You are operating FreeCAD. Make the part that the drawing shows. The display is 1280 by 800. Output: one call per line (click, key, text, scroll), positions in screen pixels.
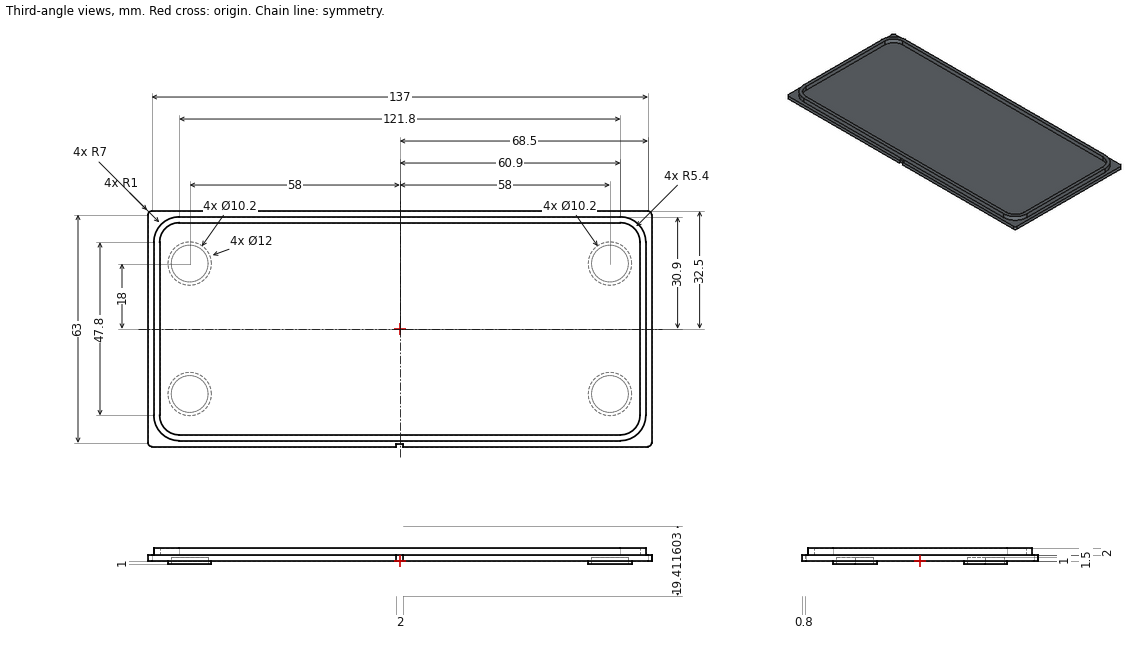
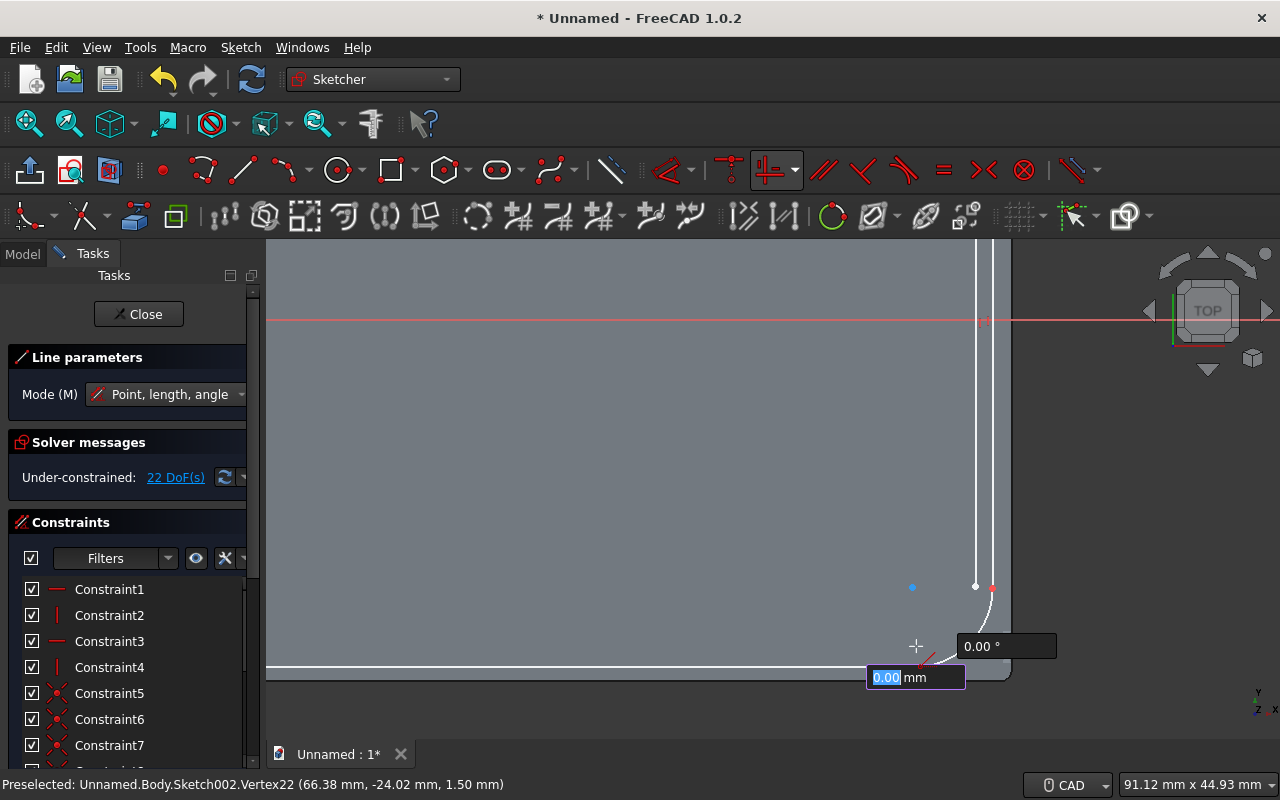
scroll(976, 588, down, 5)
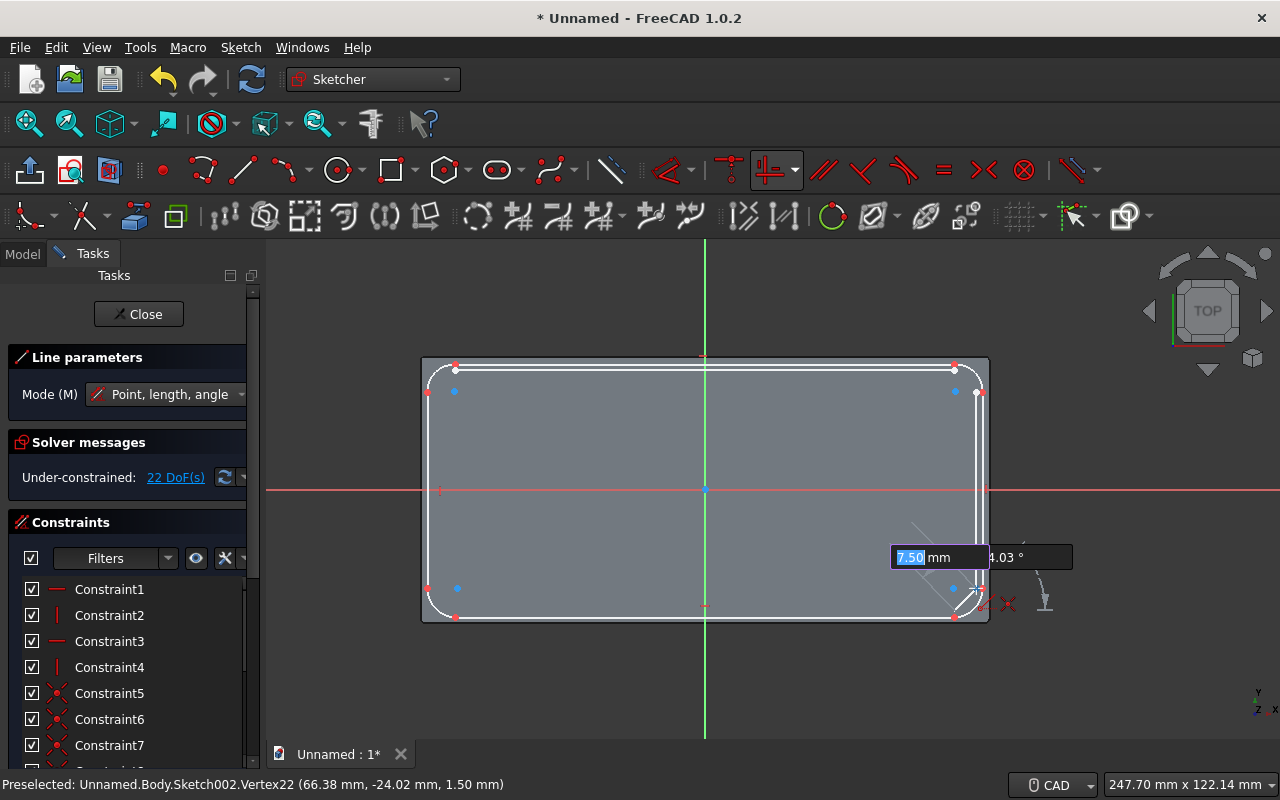
scroll(456, 610, up, 5)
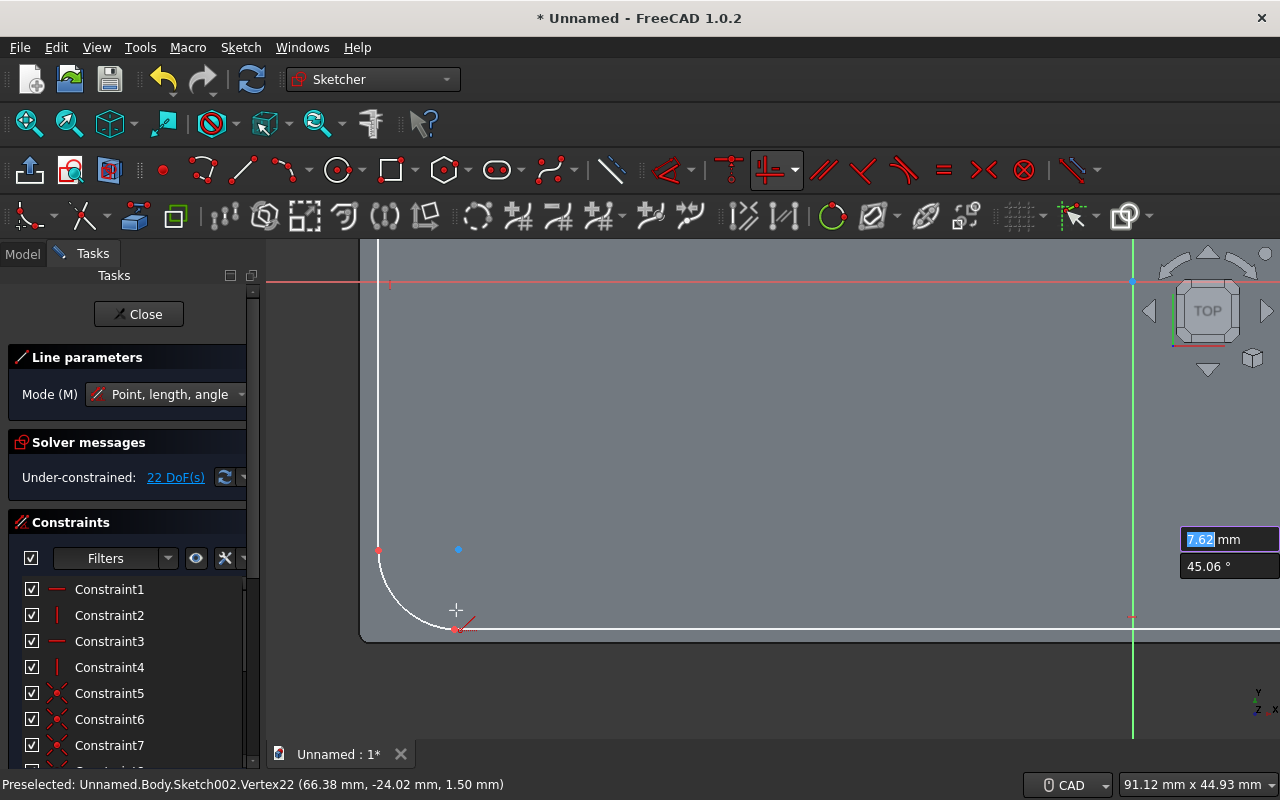
click(455, 608)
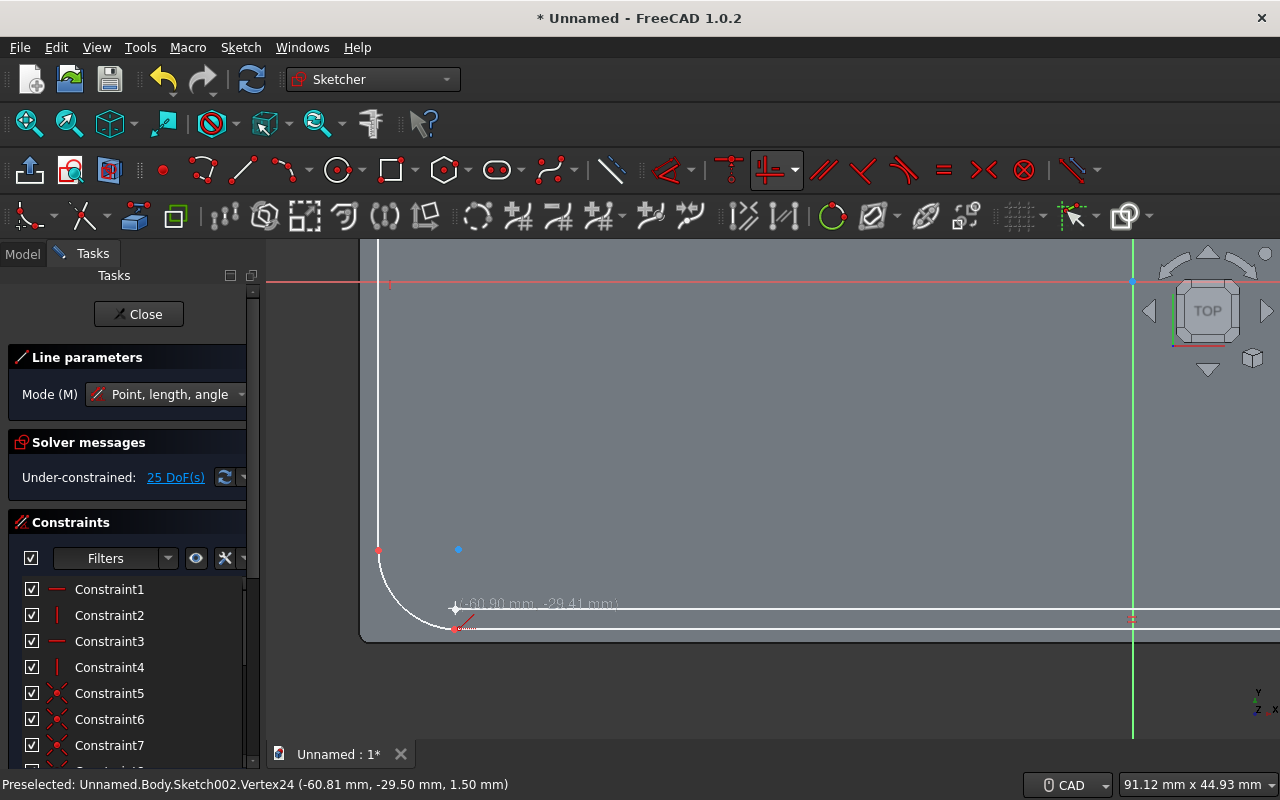
click(395, 548)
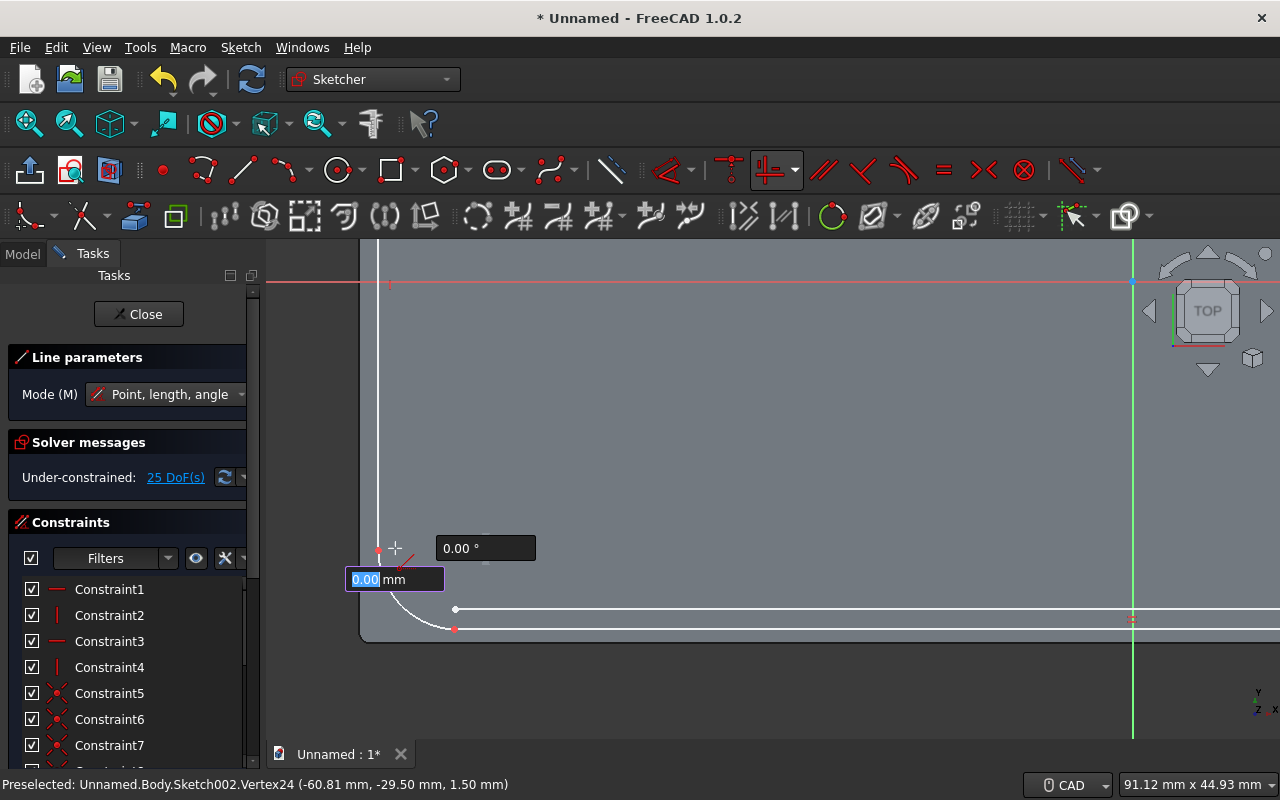
scroll(455, 610, down, 5)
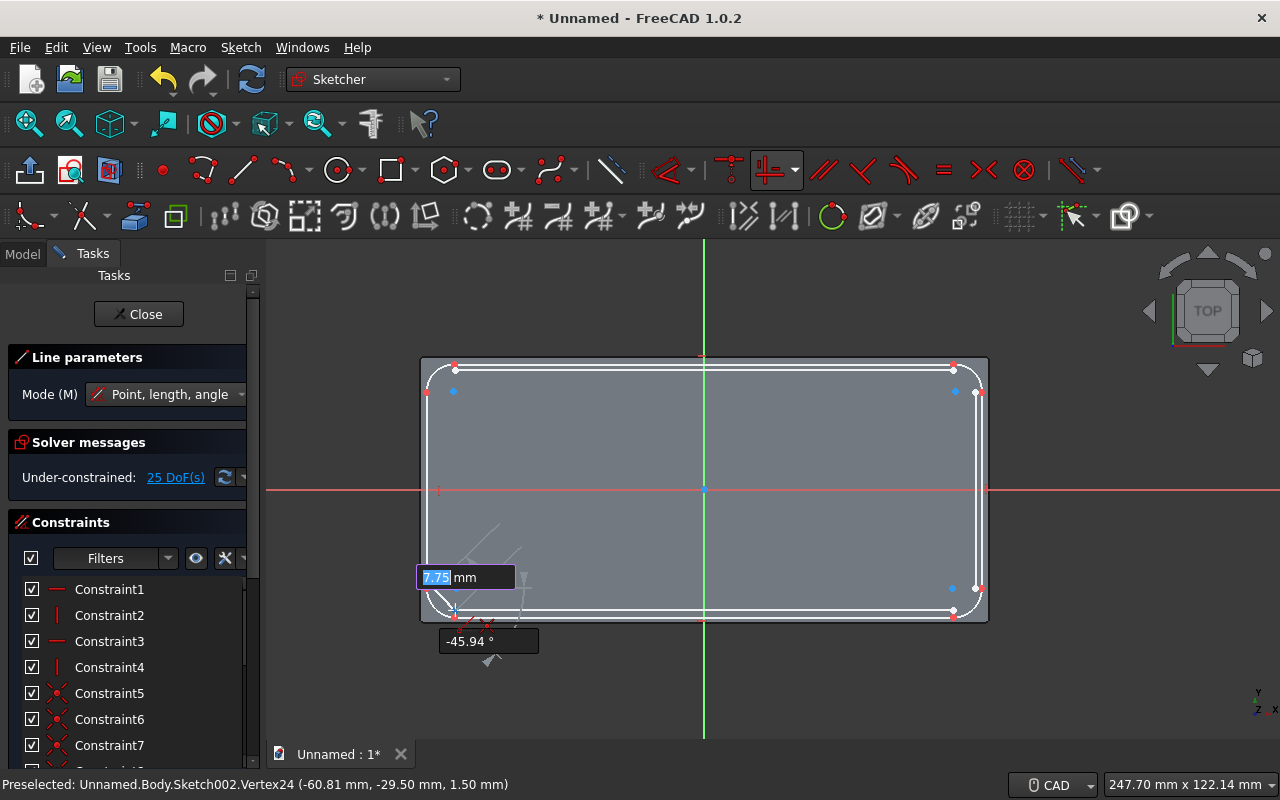
scroll(433, 392, up, 5)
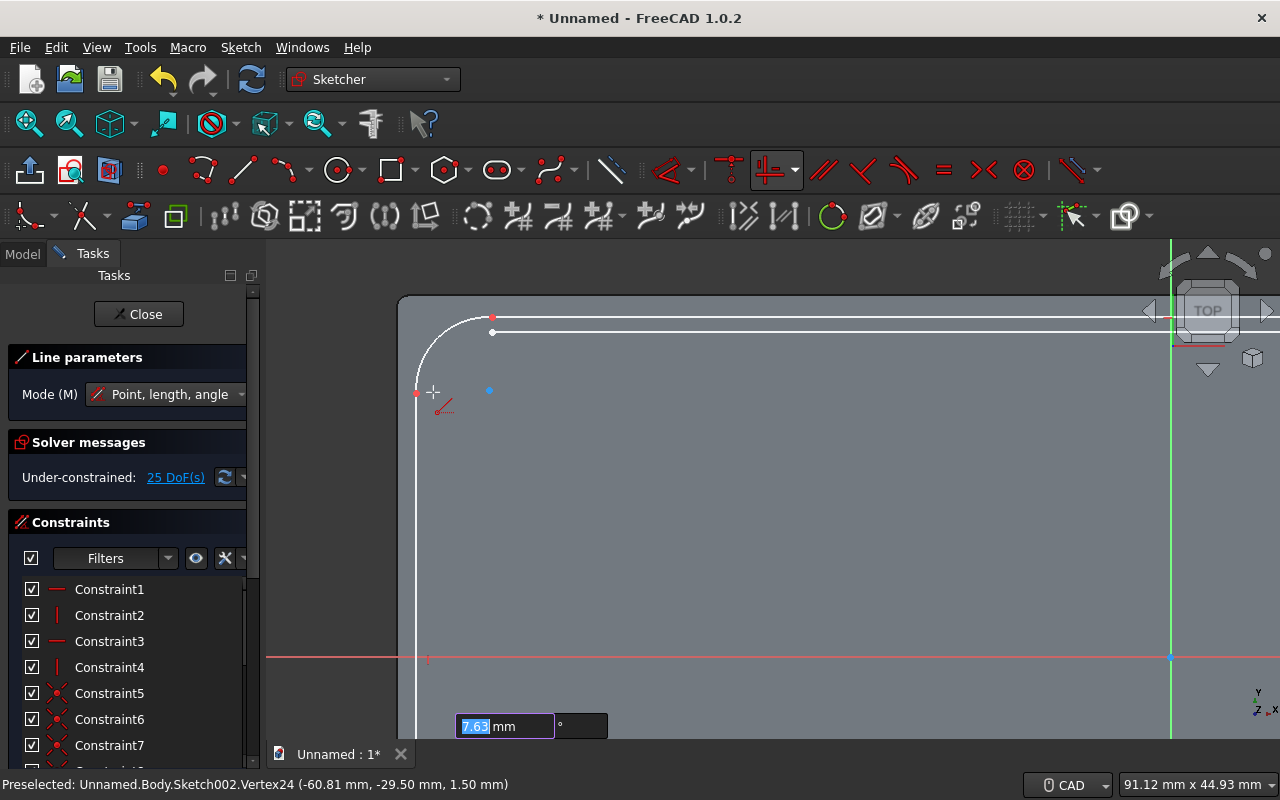
click(433, 391)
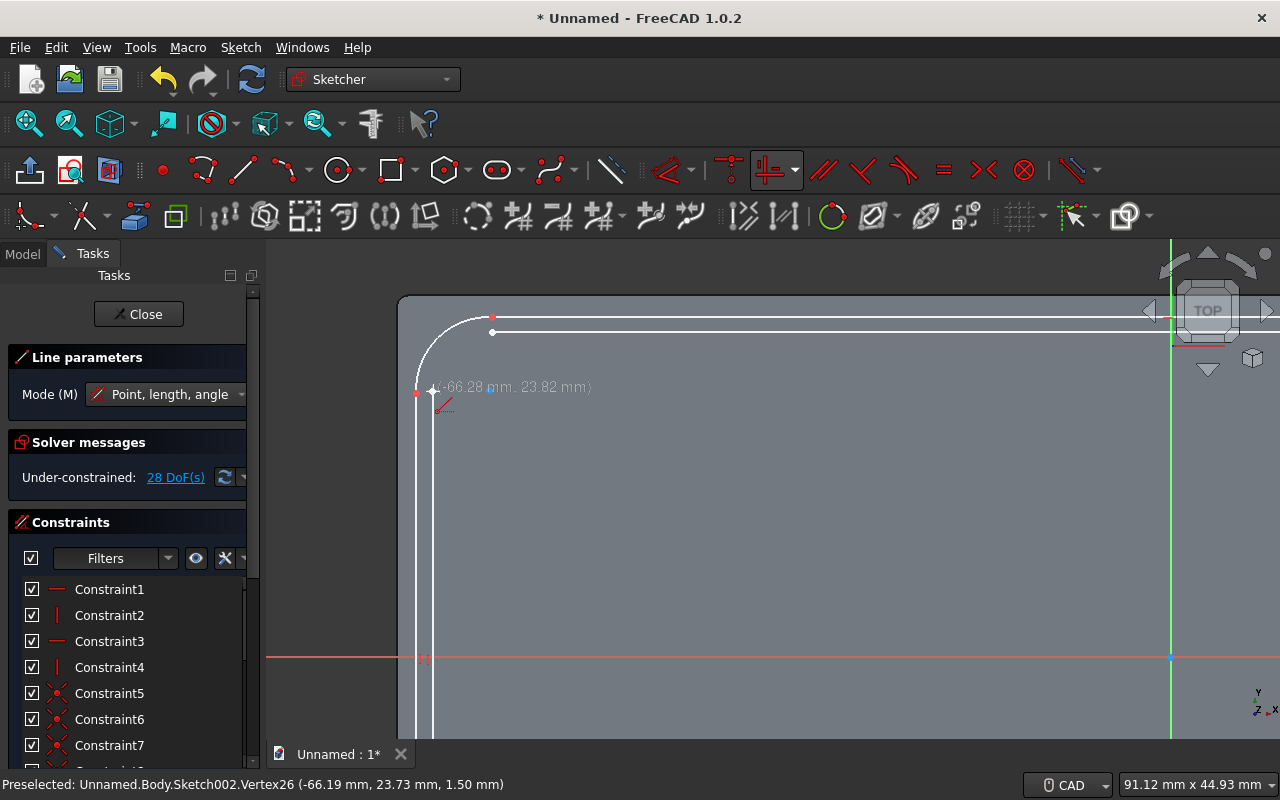
click(284, 170)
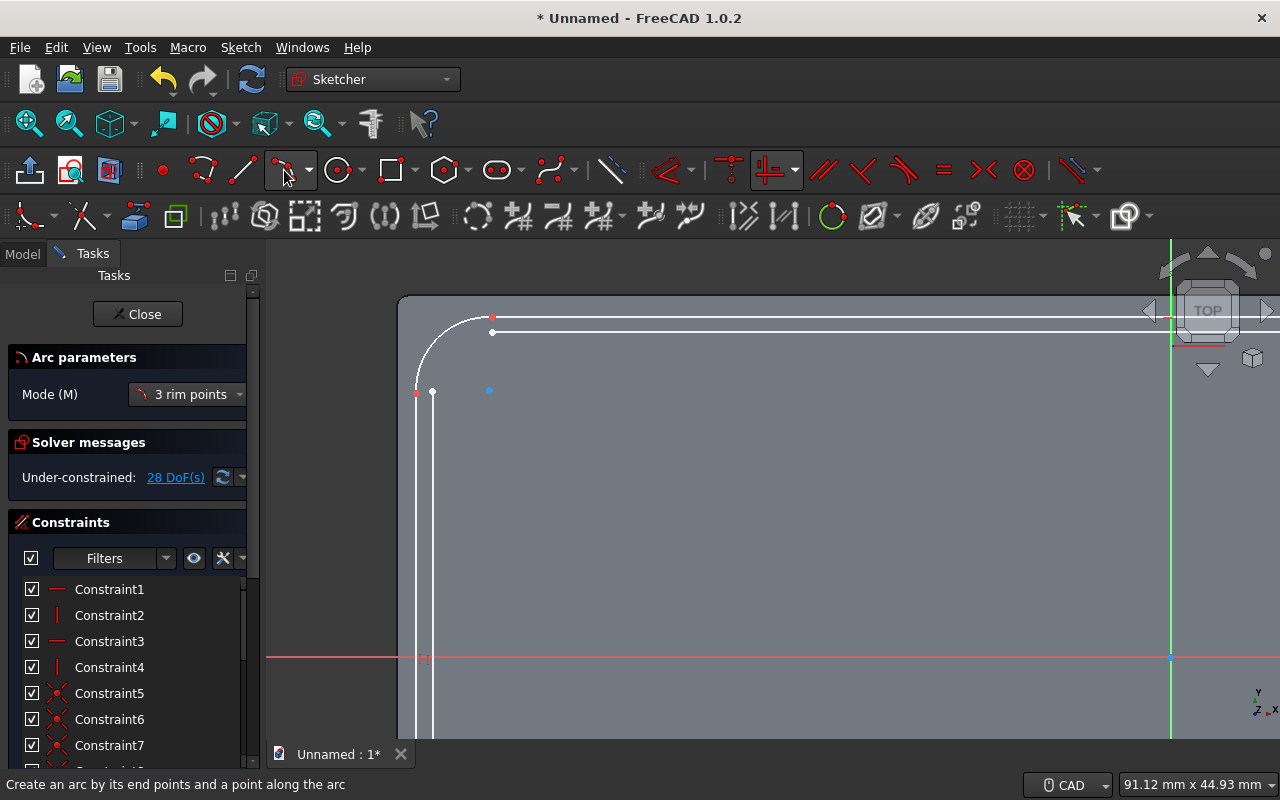
scroll(433, 391, down, 5)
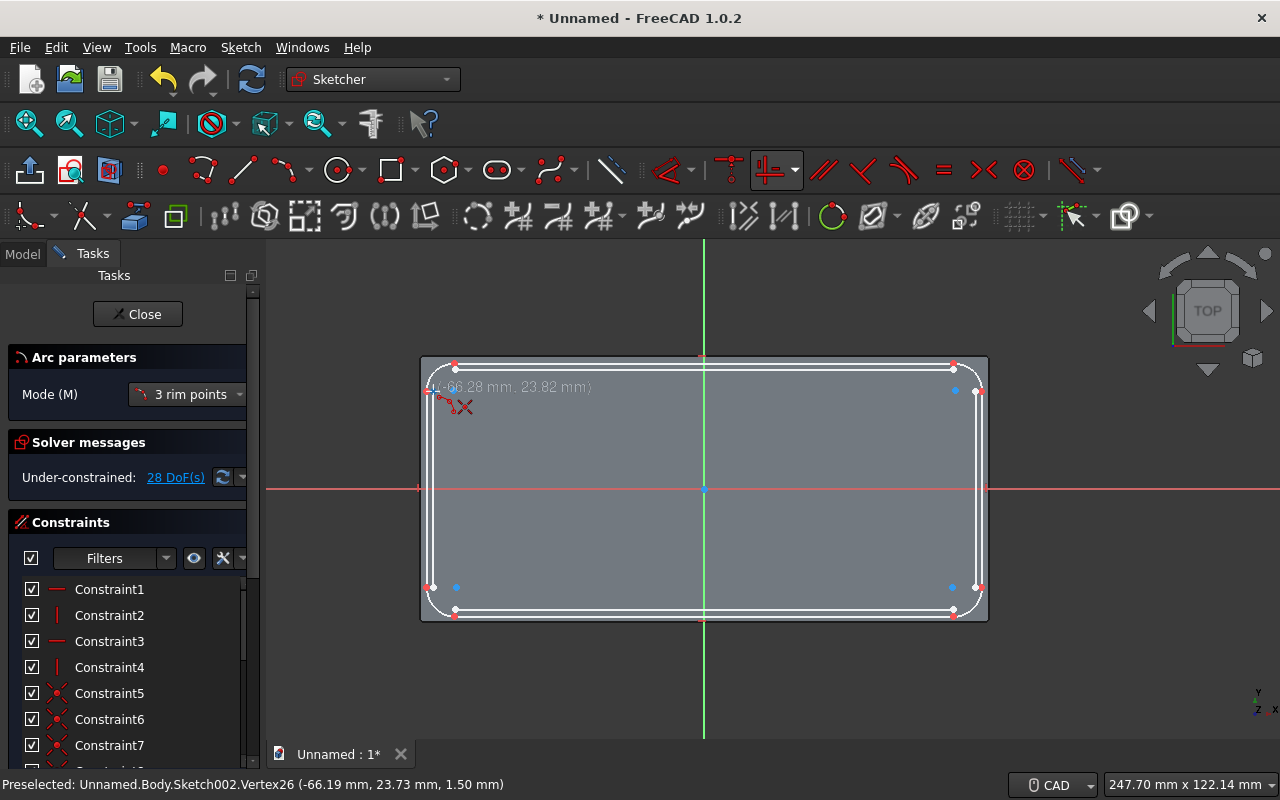
scroll(954, 369, up, 5)